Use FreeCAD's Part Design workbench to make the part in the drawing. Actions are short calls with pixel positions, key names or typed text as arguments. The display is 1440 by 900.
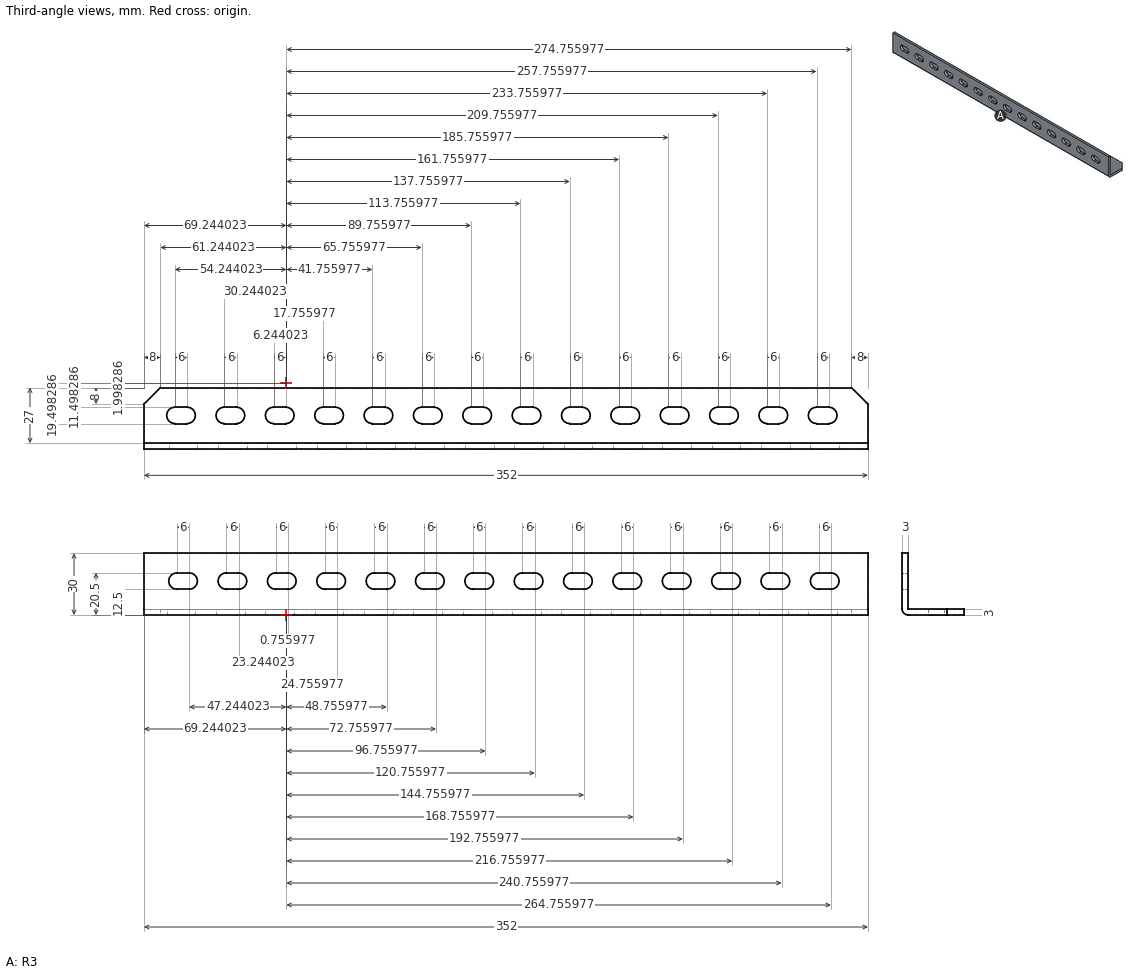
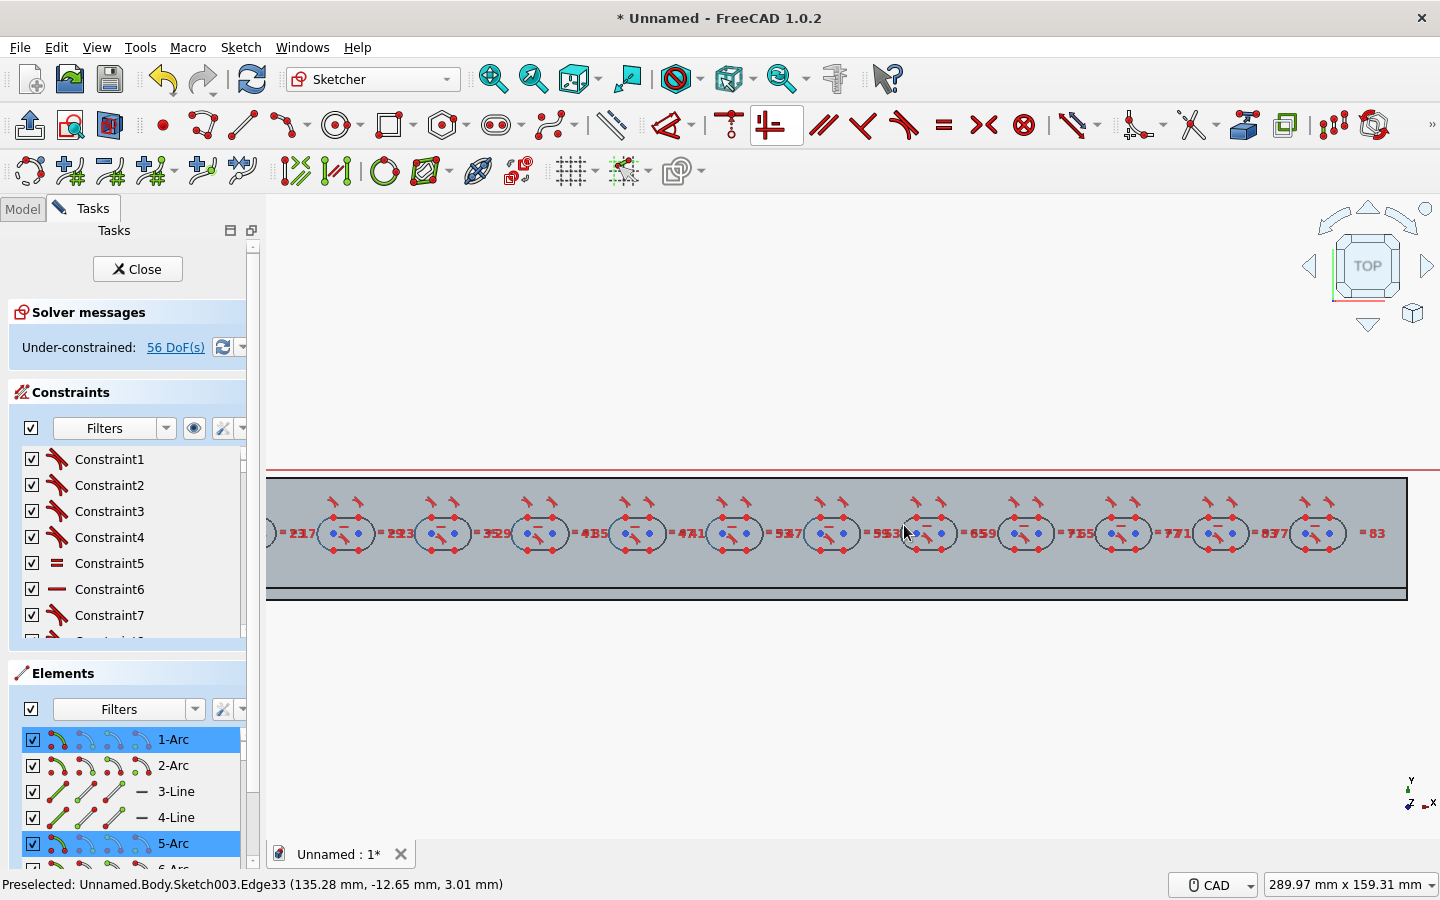
click(904, 524)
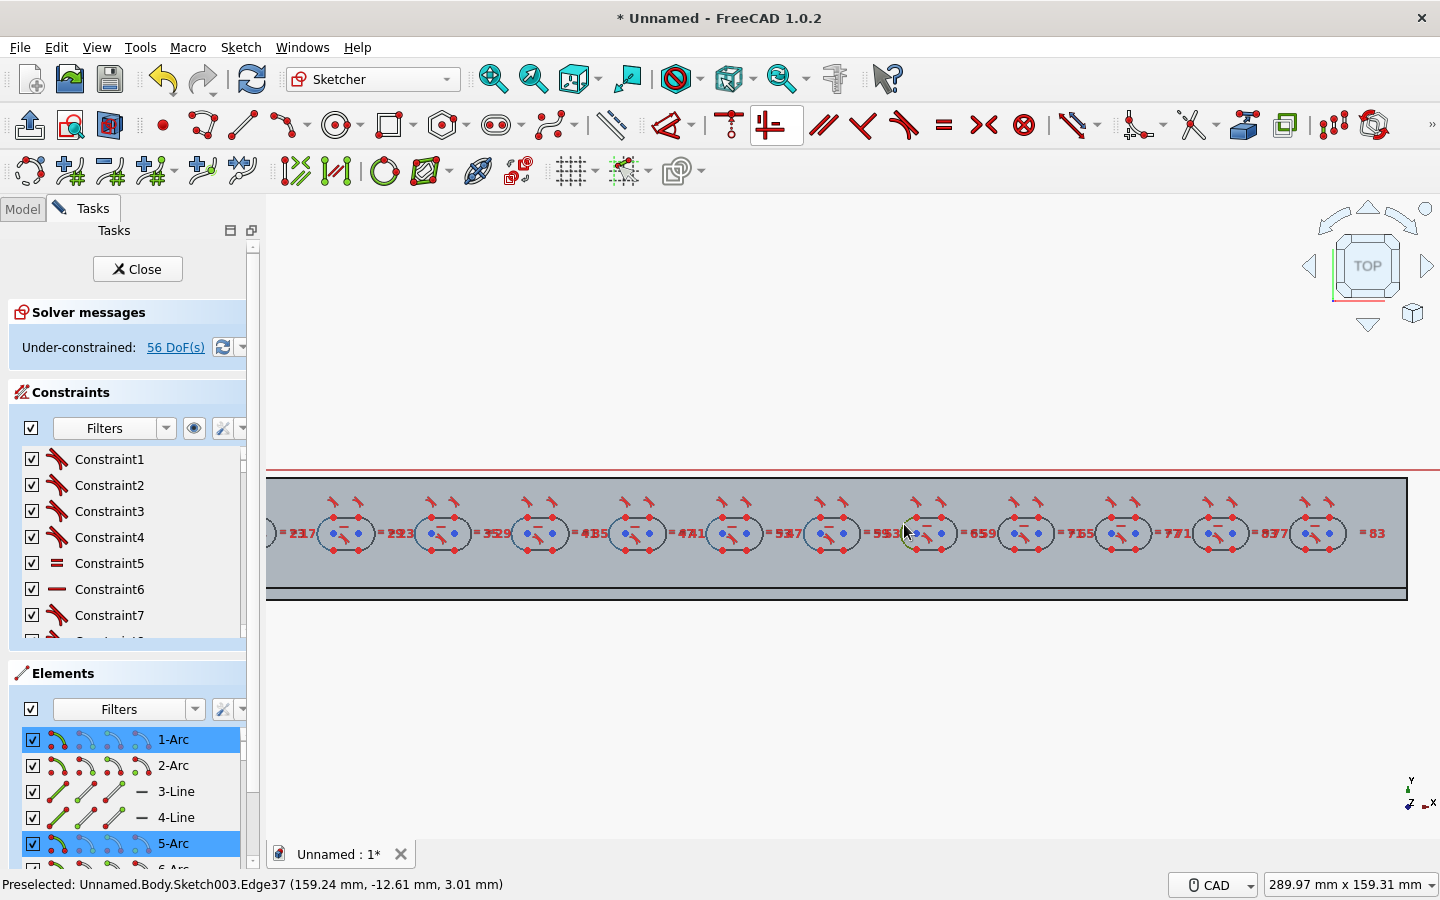
click(1001, 524)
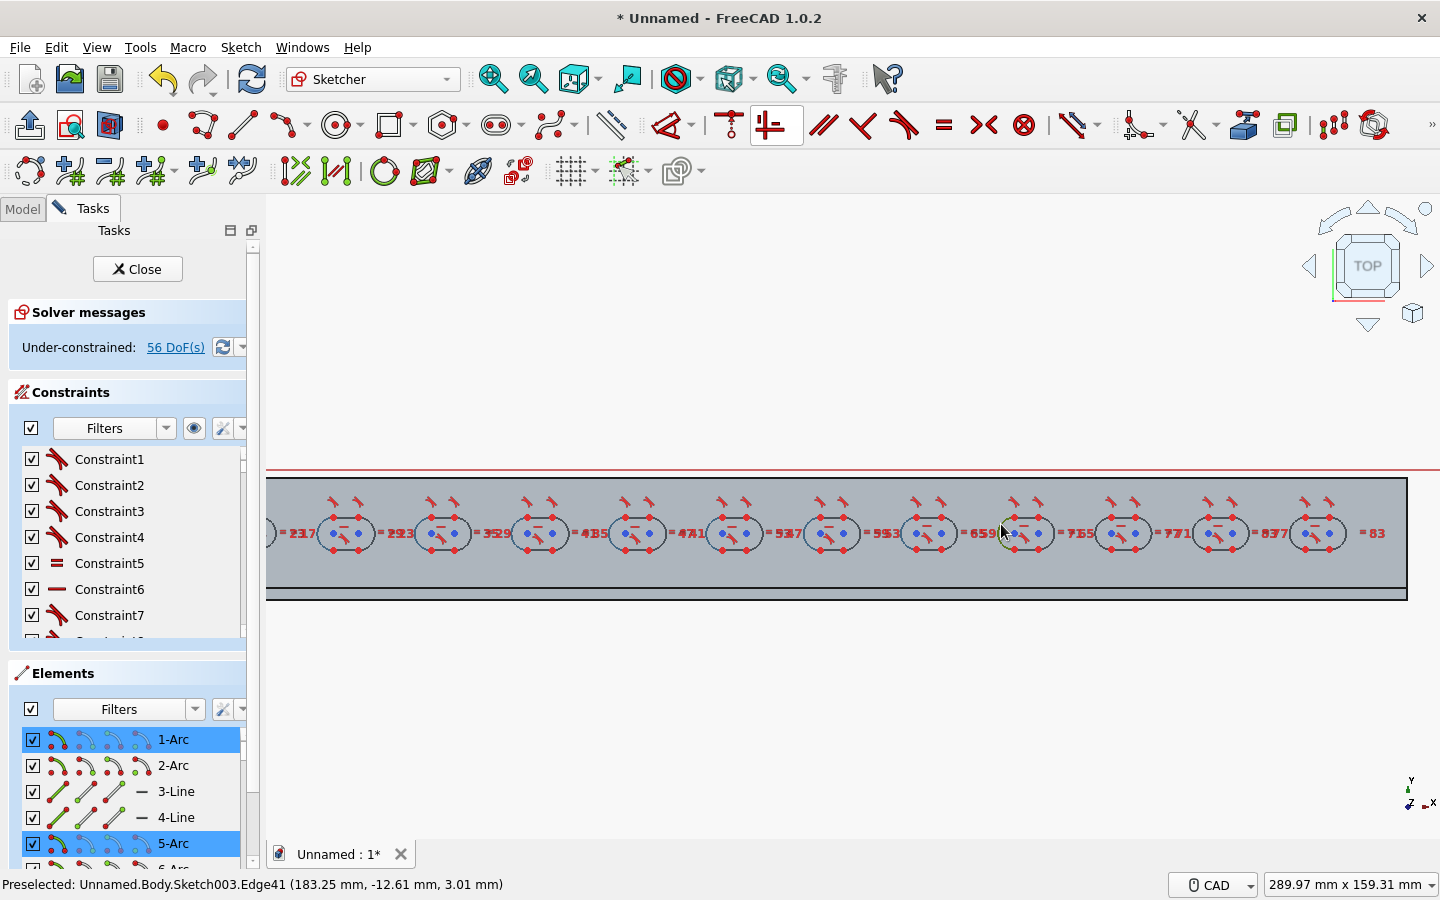
click(1098, 524)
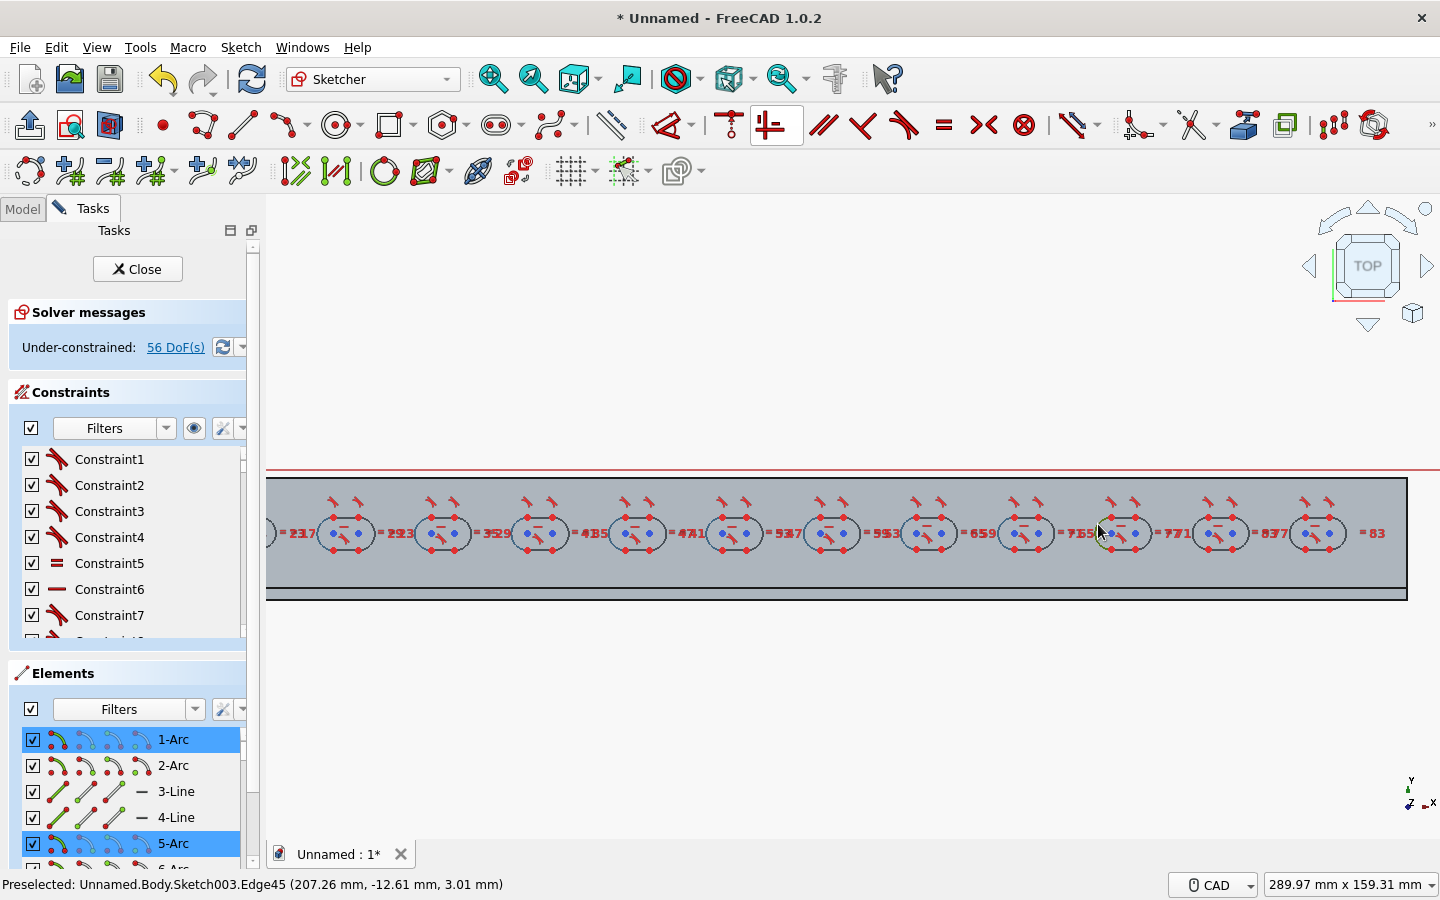
click(1196, 524)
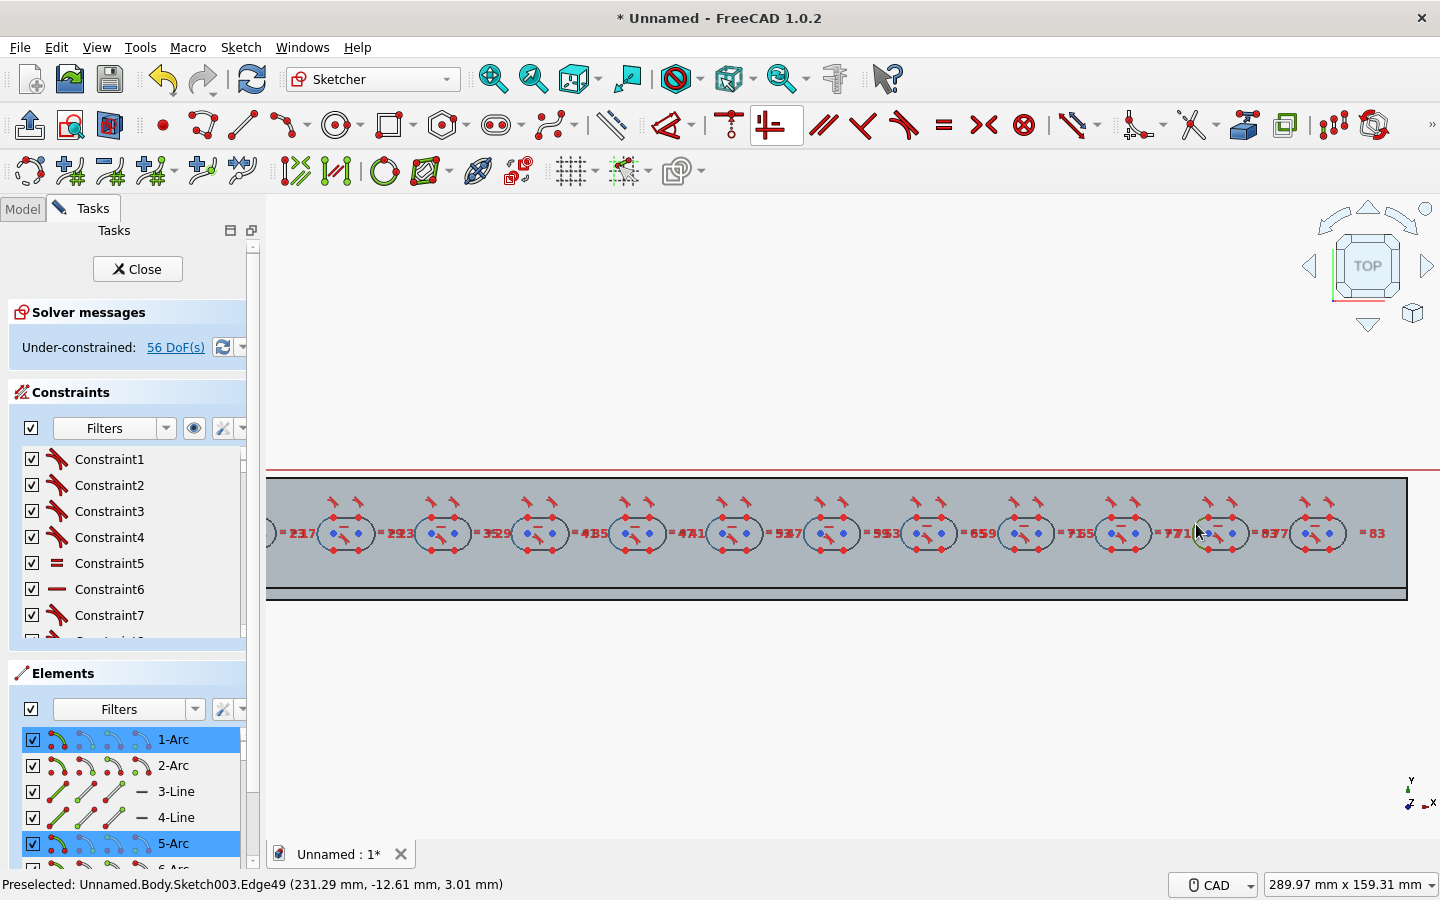
scroll(904, 525, down, 3)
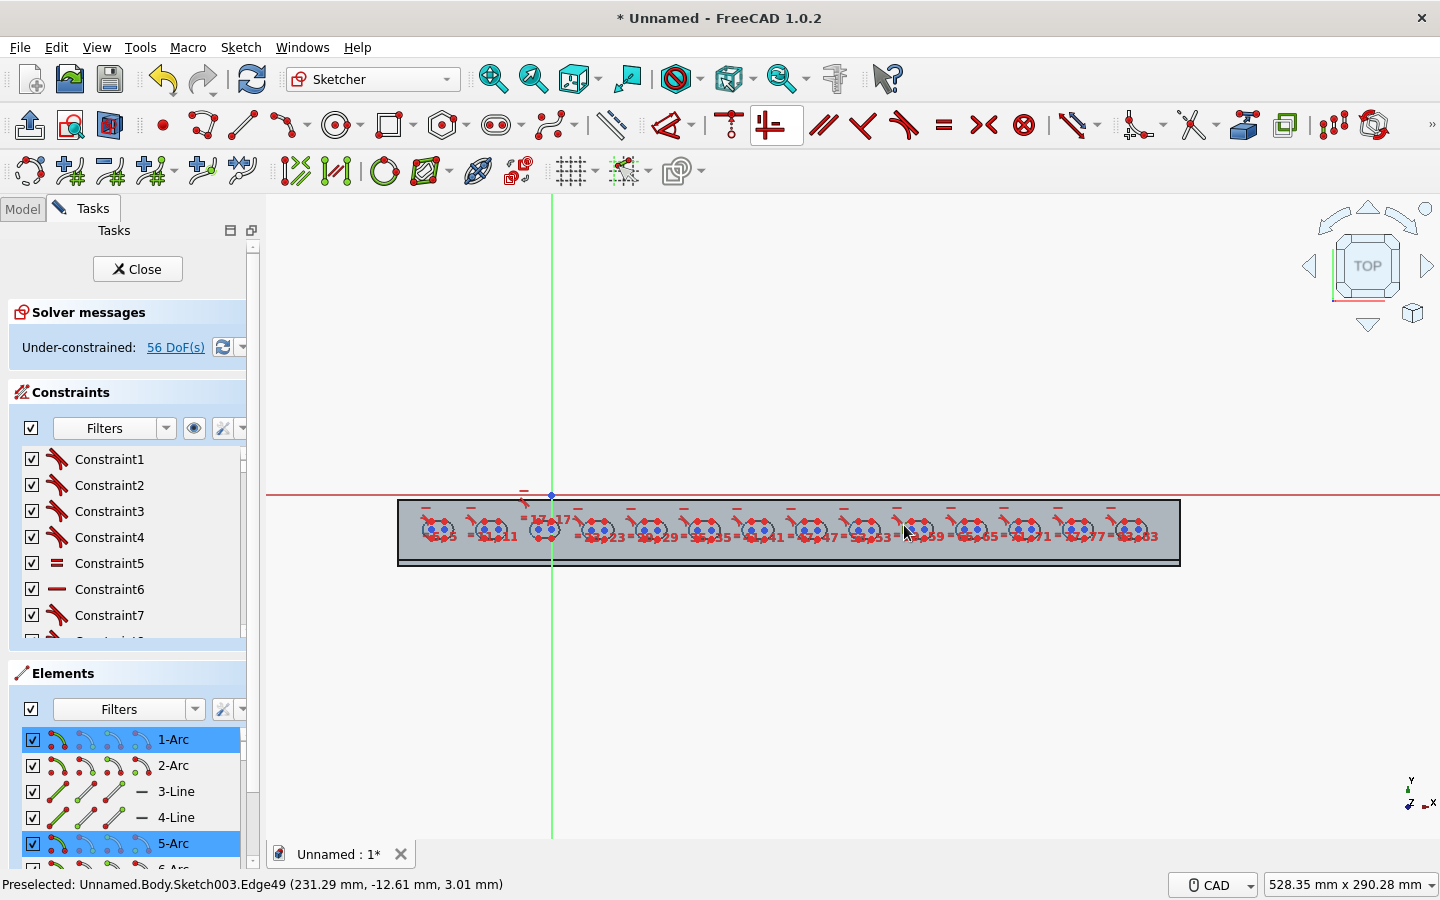
scroll(1118, 525, up, 3)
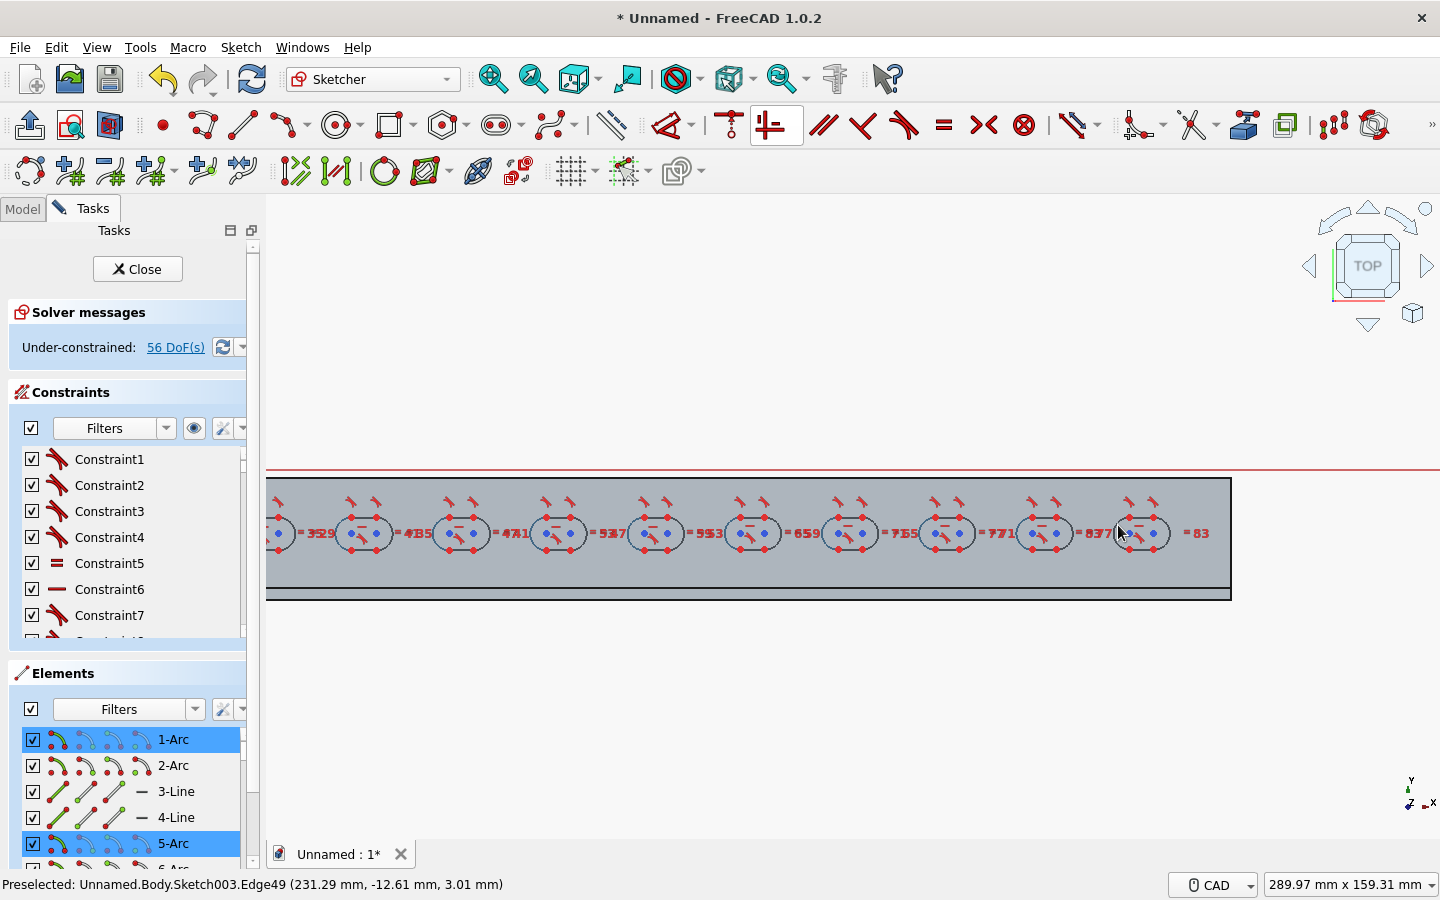
click(1117, 524)